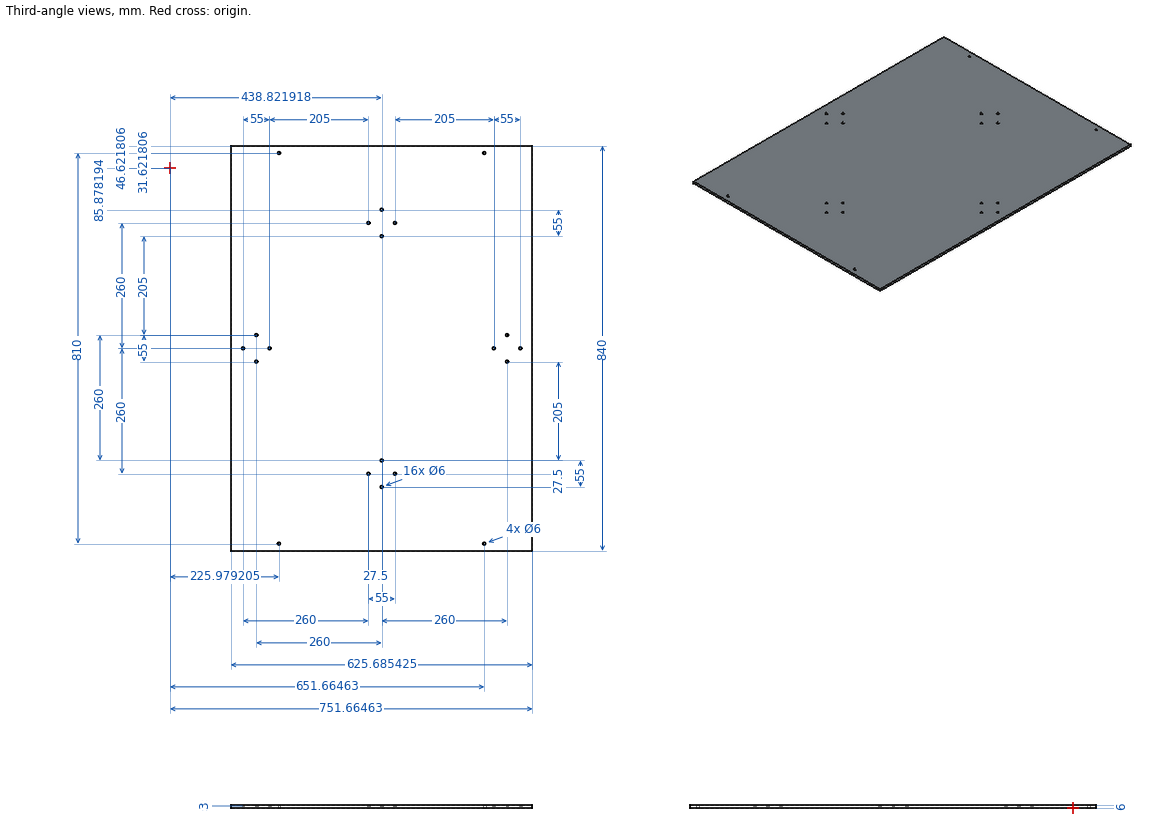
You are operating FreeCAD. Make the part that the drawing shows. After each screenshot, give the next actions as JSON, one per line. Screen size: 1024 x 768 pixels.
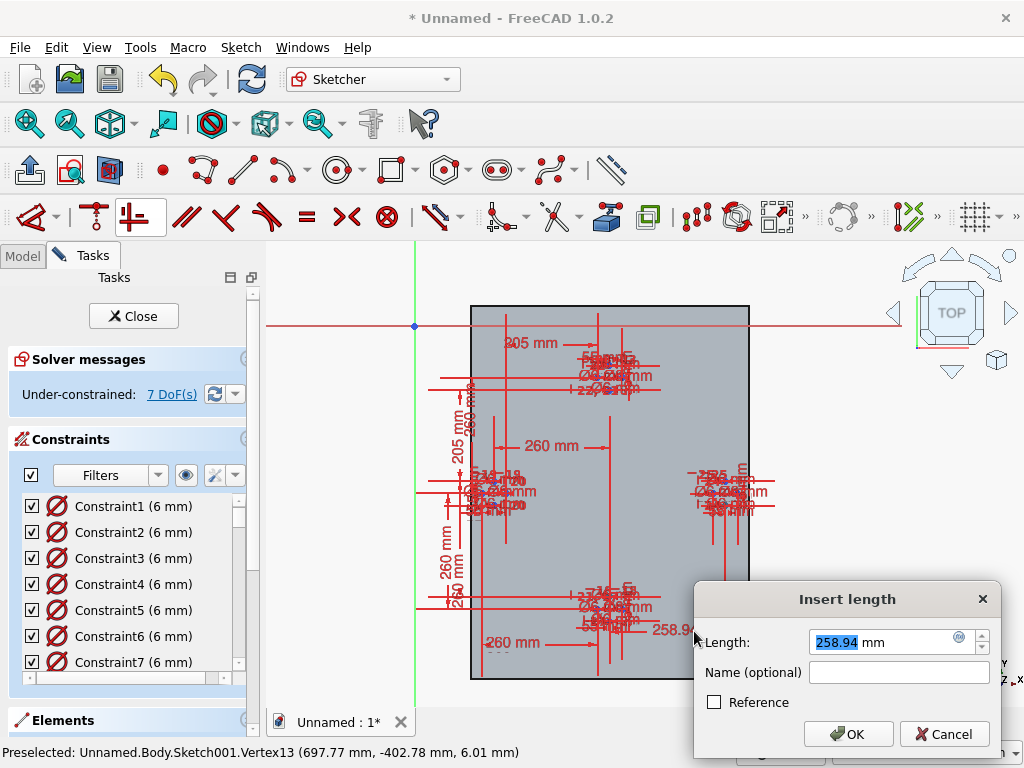
{"action": "type", "text": "260"}
{"action": "key", "text": "Return"}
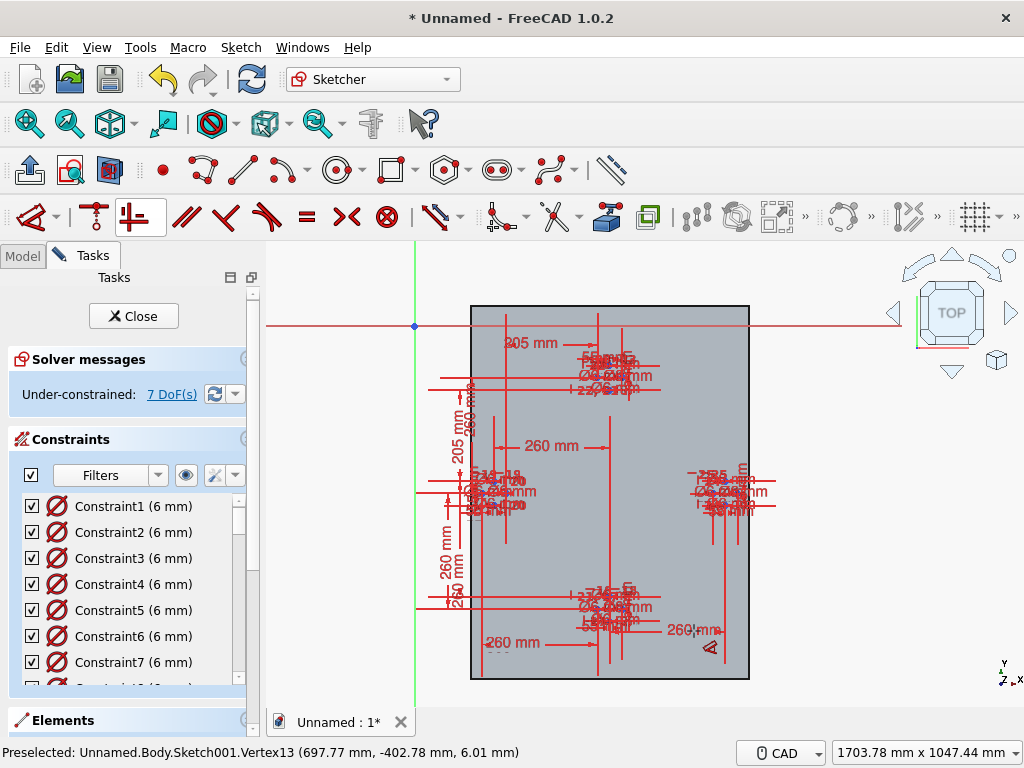
{"action": "left_click", "coordinate": [610, 597]}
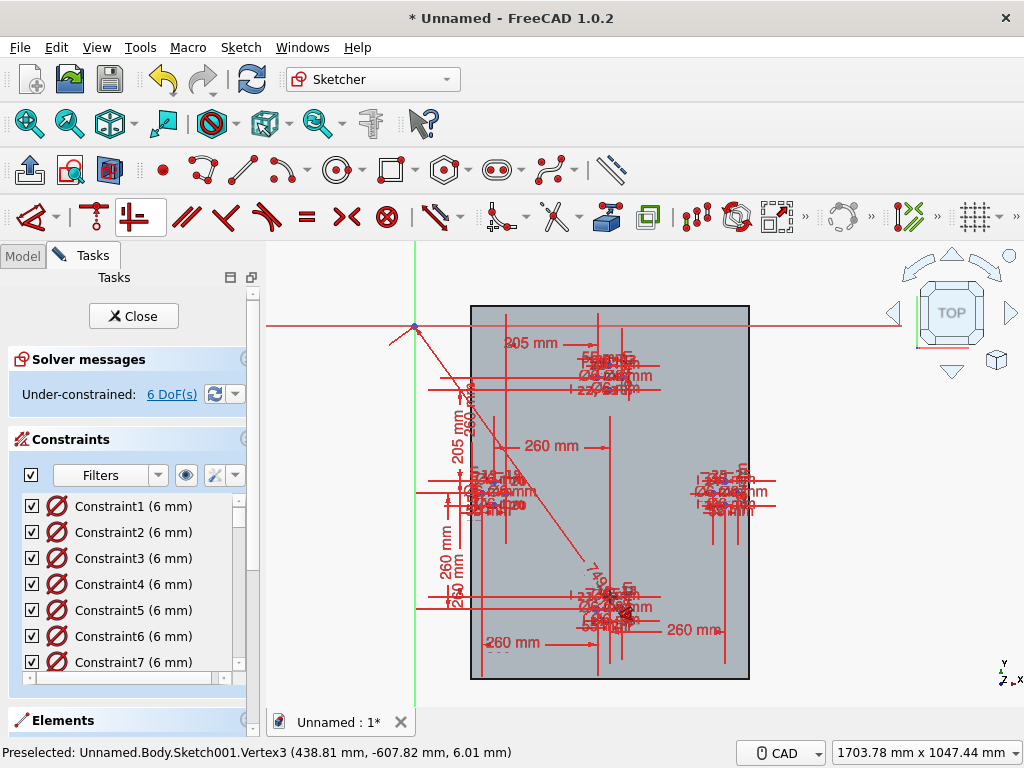
{"action": "left_click", "coordinate": [725, 506]}
{"action": "left_click", "coordinate": [759, 551]}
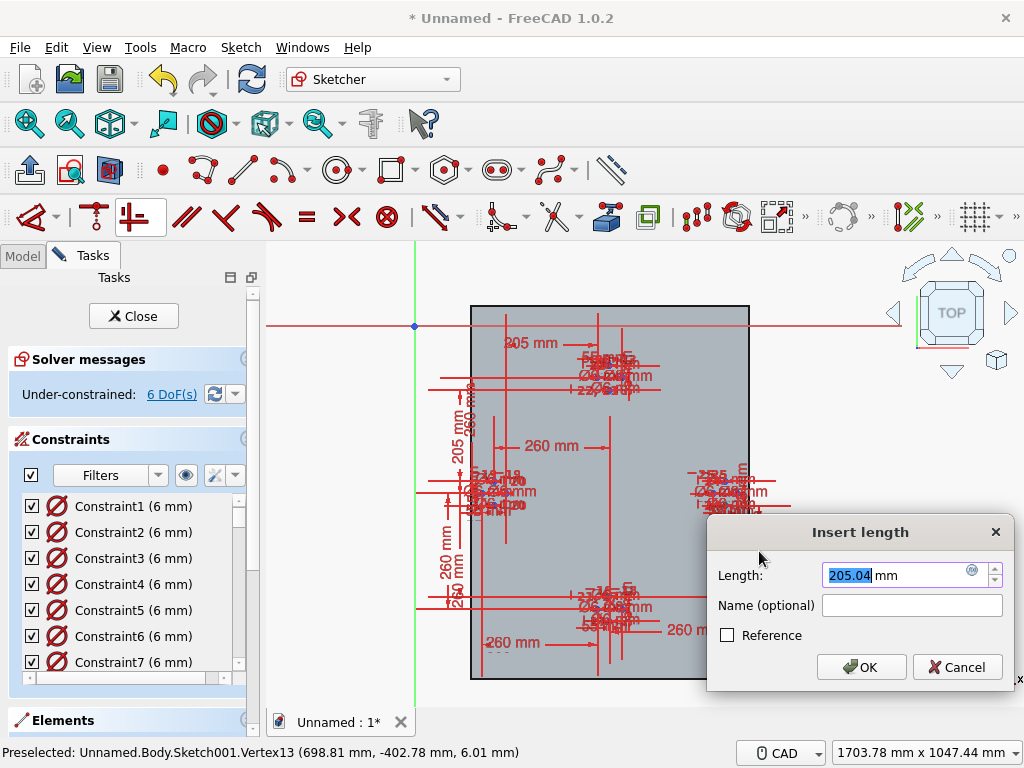
{"action": "type", "text": "205"}
{"action": "key", "text": "Return"}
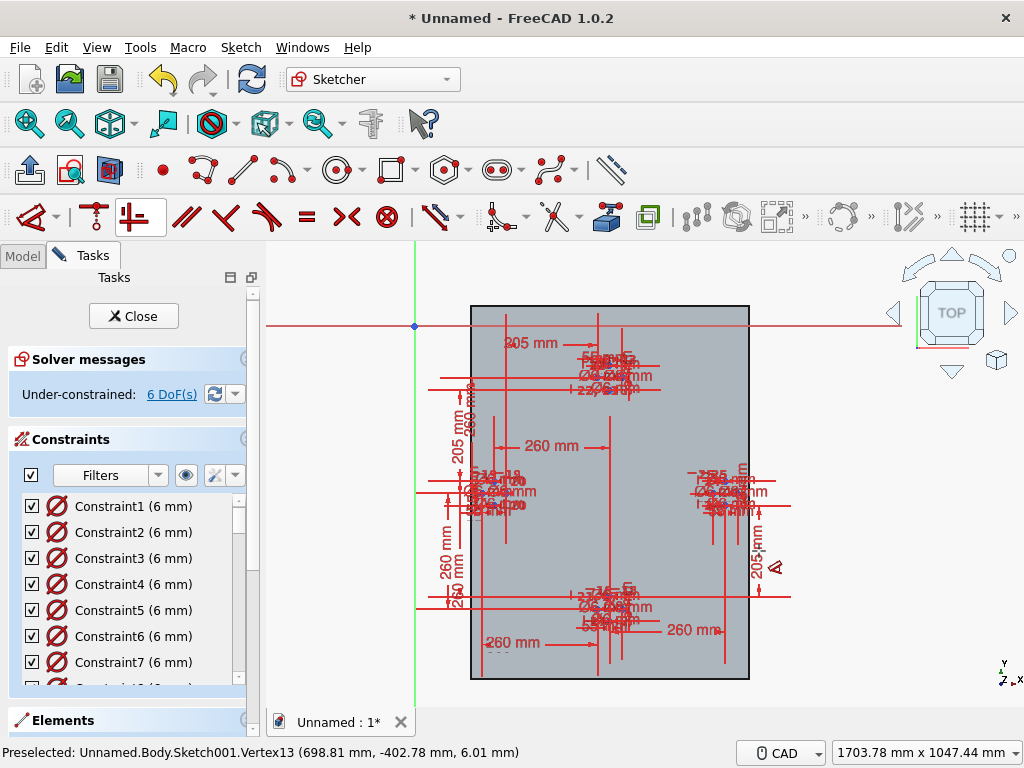
{"action": "left_click", "coordinate": [622, 378]}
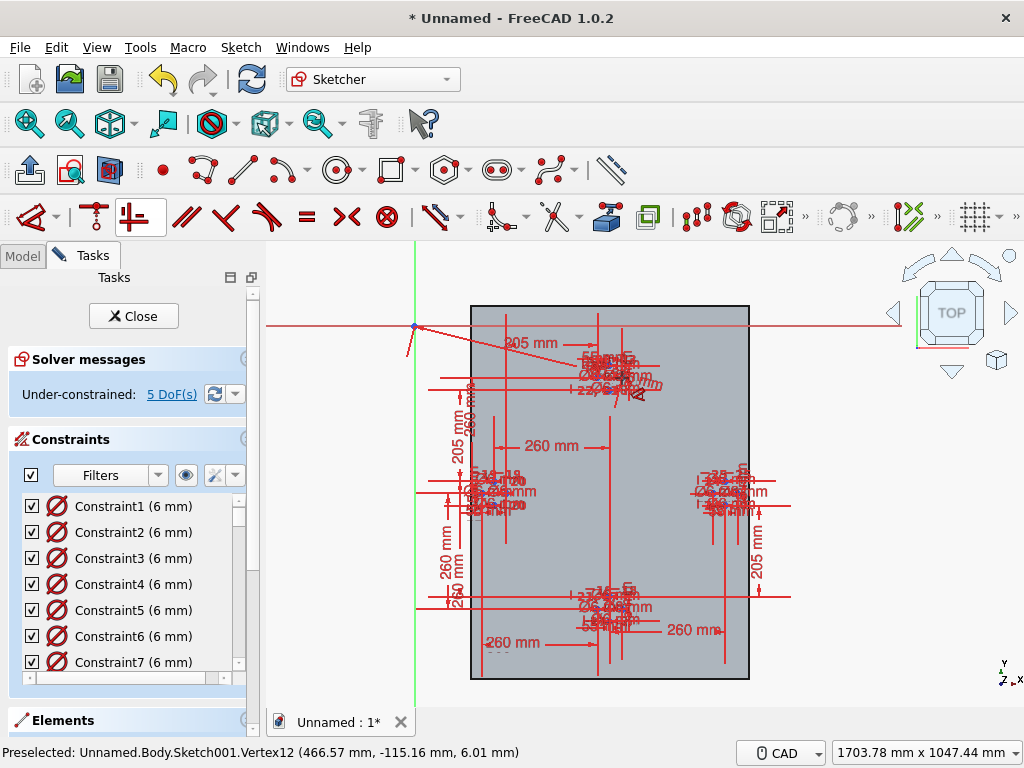
{"action": "left_click", "coordinate": [713, 494]}
{"action": "left_click", "coordinate": [689, 344]}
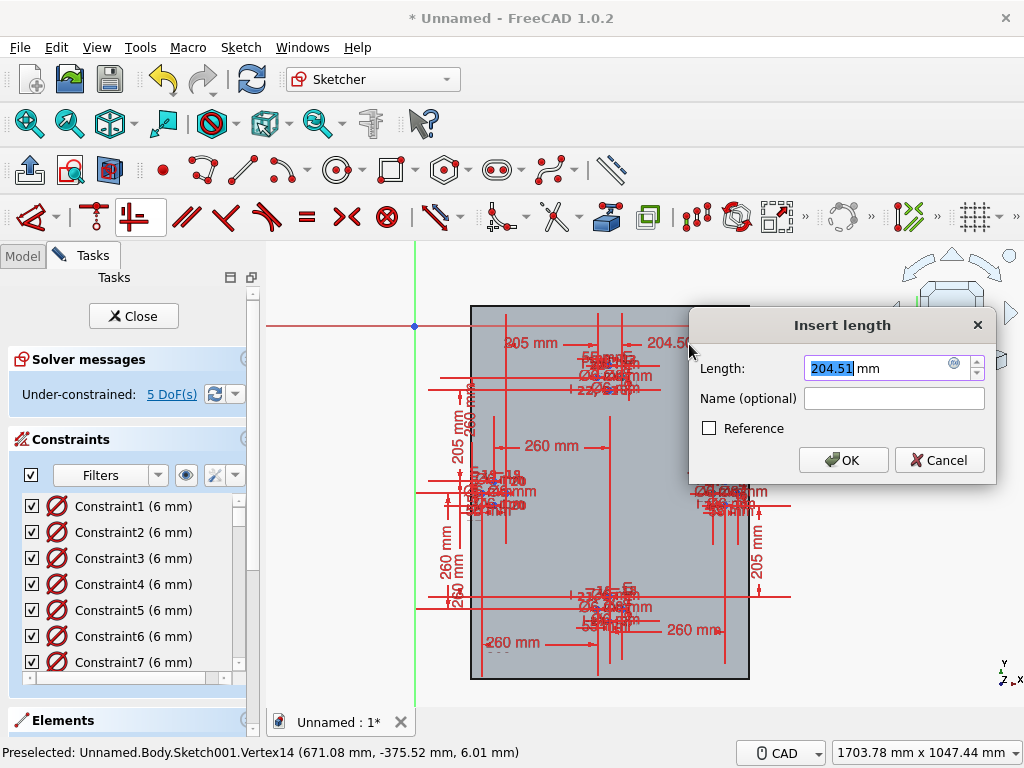
{"action": "type", "text": "205"}
{"action": "key", "text": "Return"}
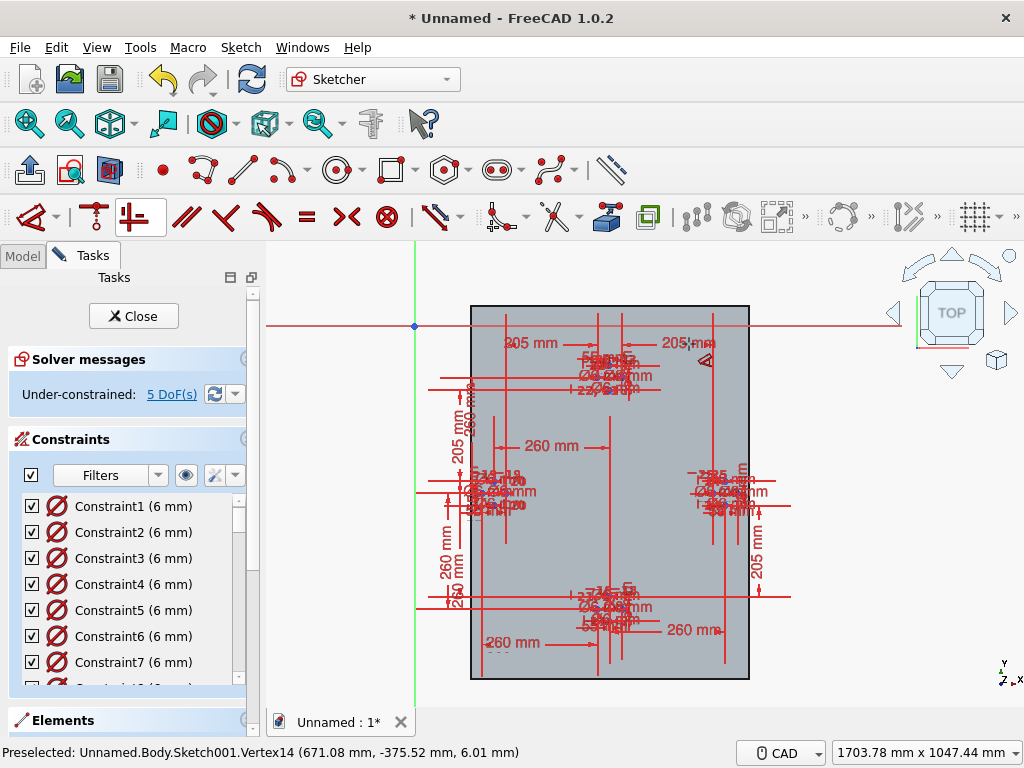
{"action": "left_click", "coordinate": [622, 378]}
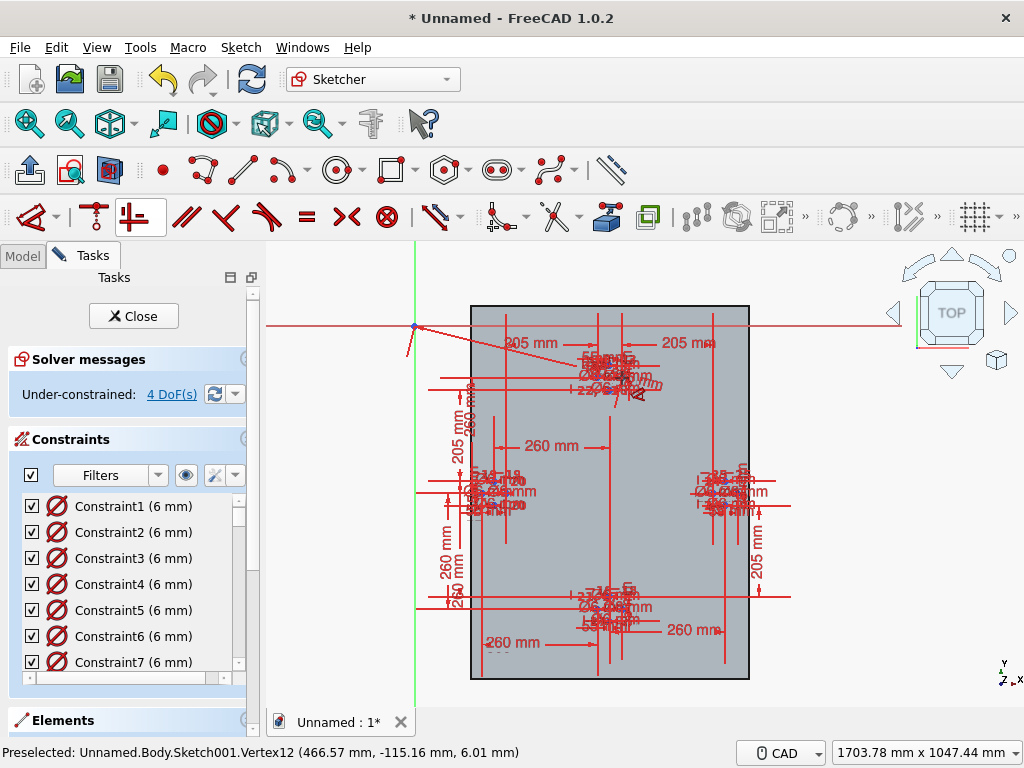
{"action": "left_click", "coordinate": [713, 494]}
{"action": "left_click", "coordinate": [747, 436]}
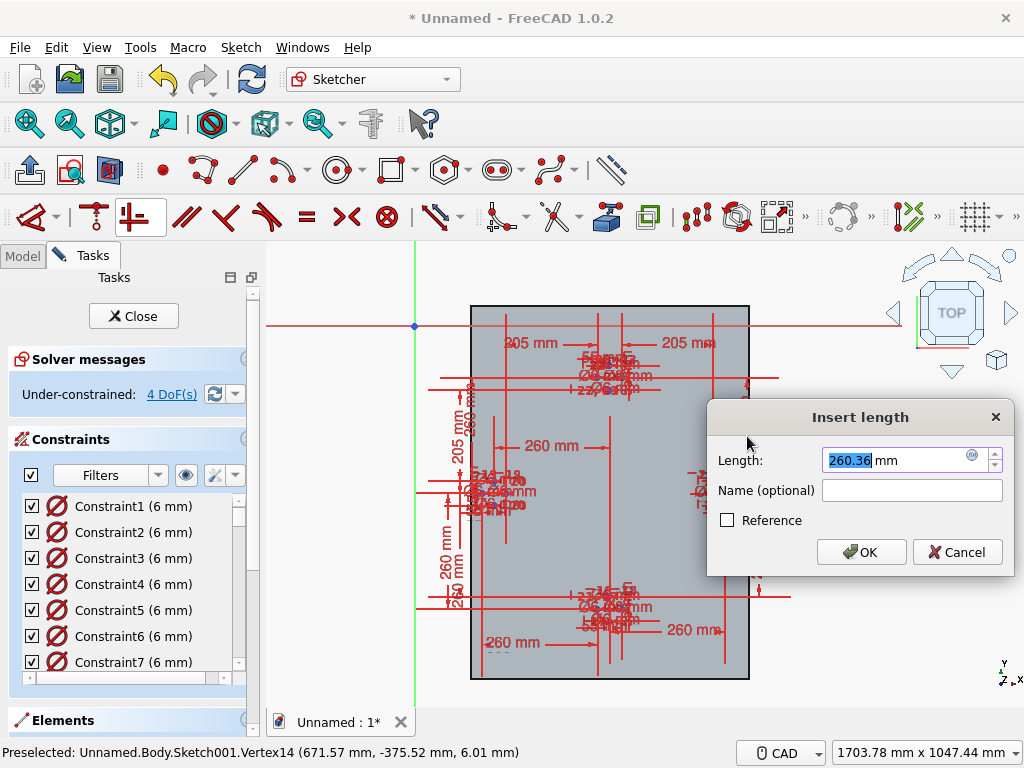
{"action": "type", "text": "260"}
{"action": "key", "text": "Return"}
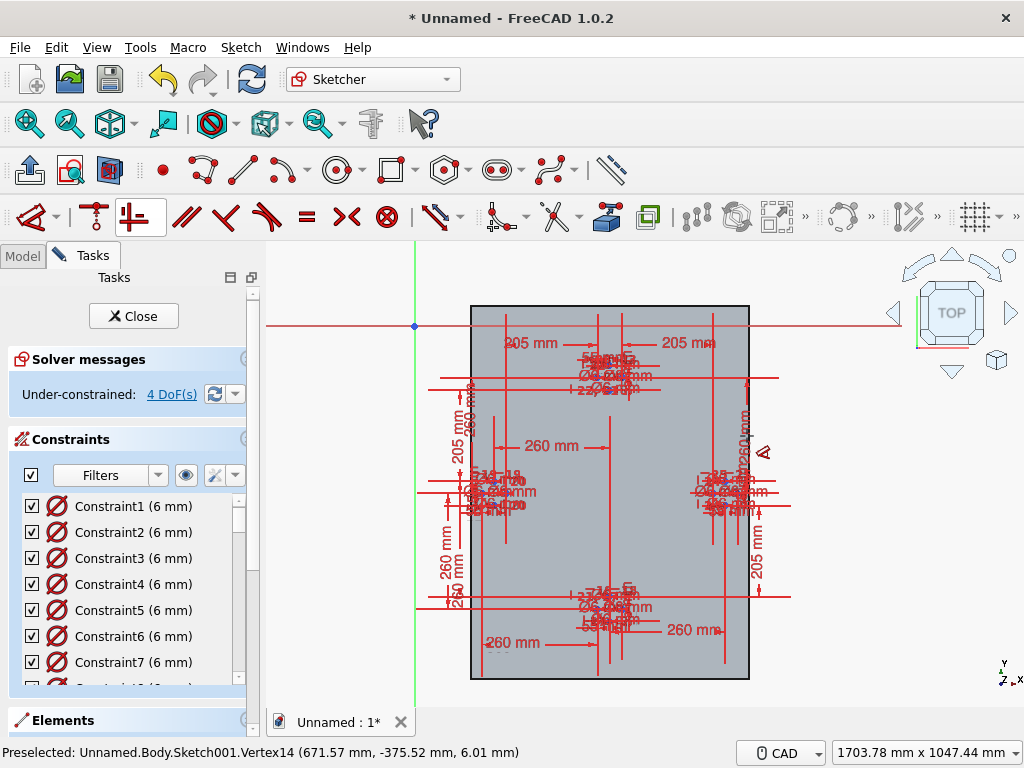
{"action": "scroll", "coordinate": [610, 621], "scroll_direction": "up", "scroll_amount": 6}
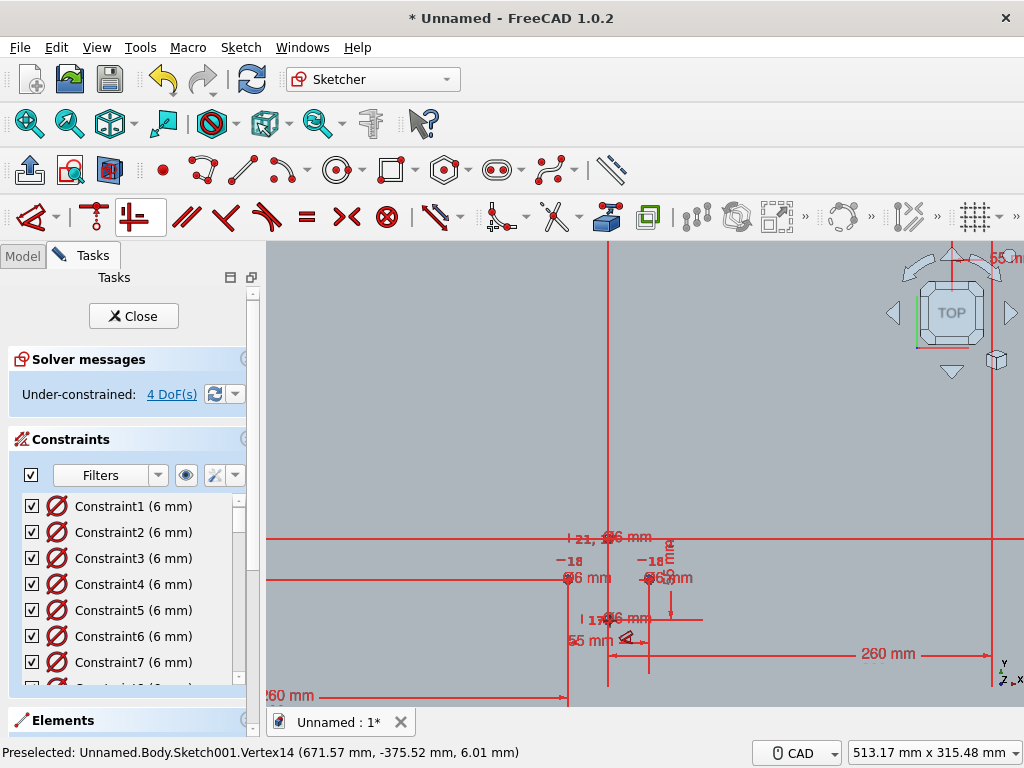
{"action": "left_click", "coordinate": [608, 620]}